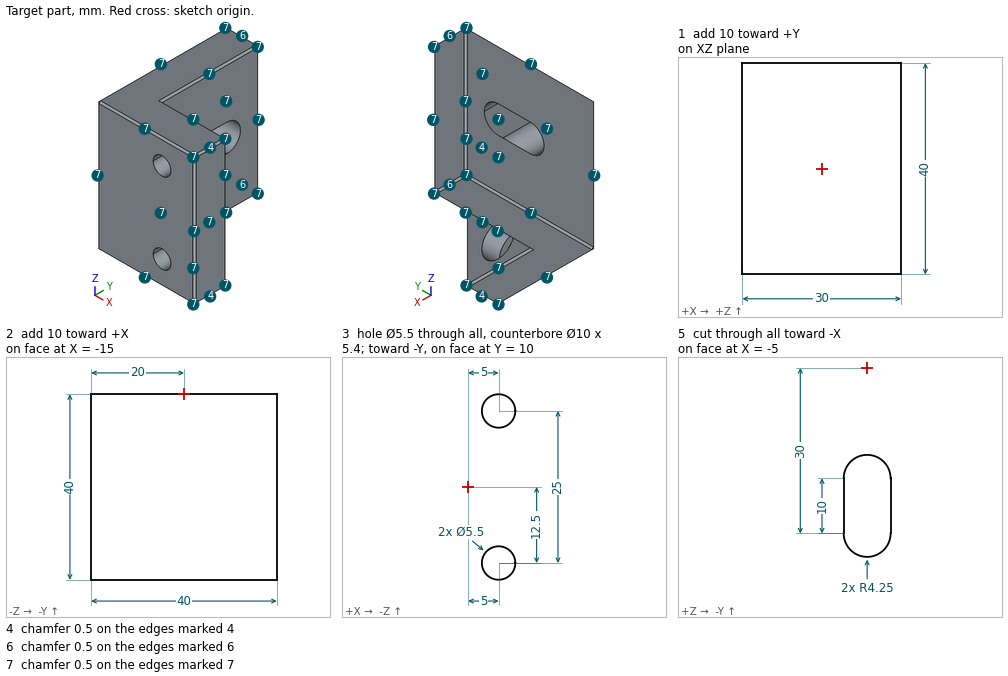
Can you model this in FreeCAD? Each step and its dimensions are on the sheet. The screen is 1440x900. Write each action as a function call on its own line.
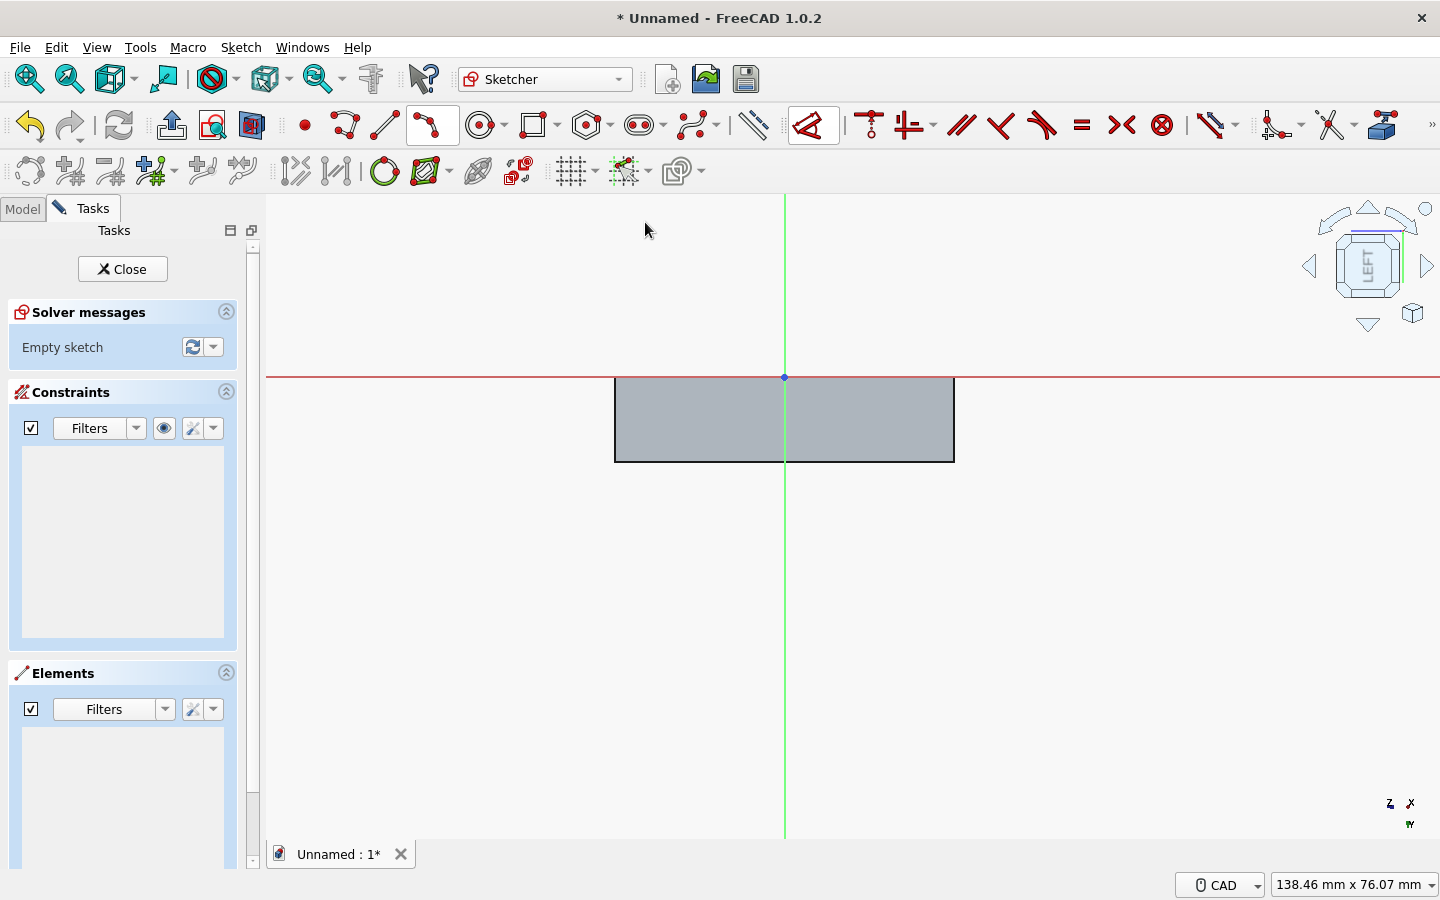
click(534, 126)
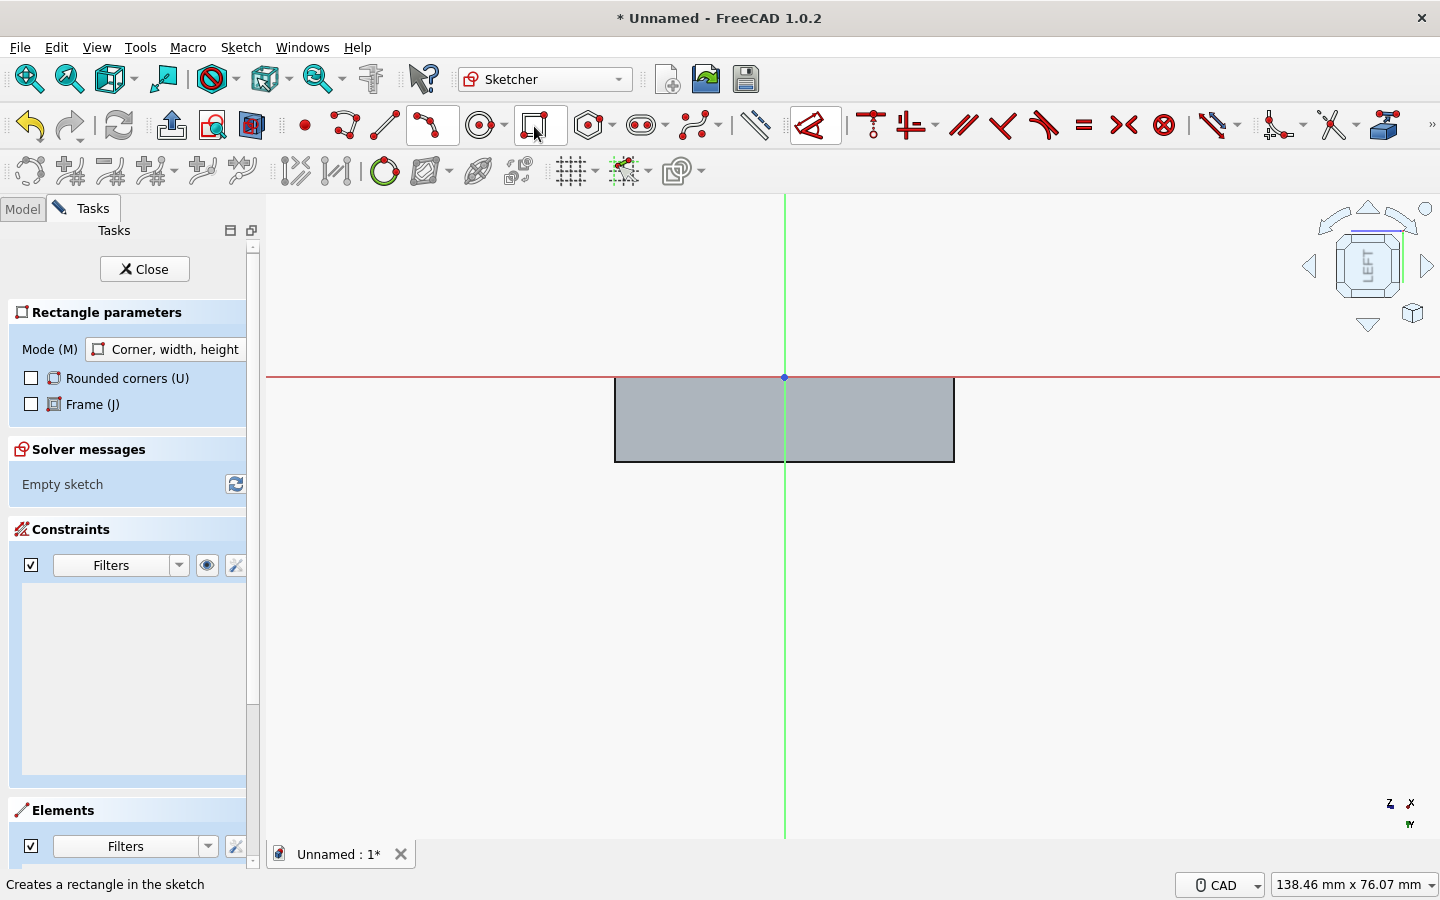
click(615, 377)
click(954, 716)
key(Escape)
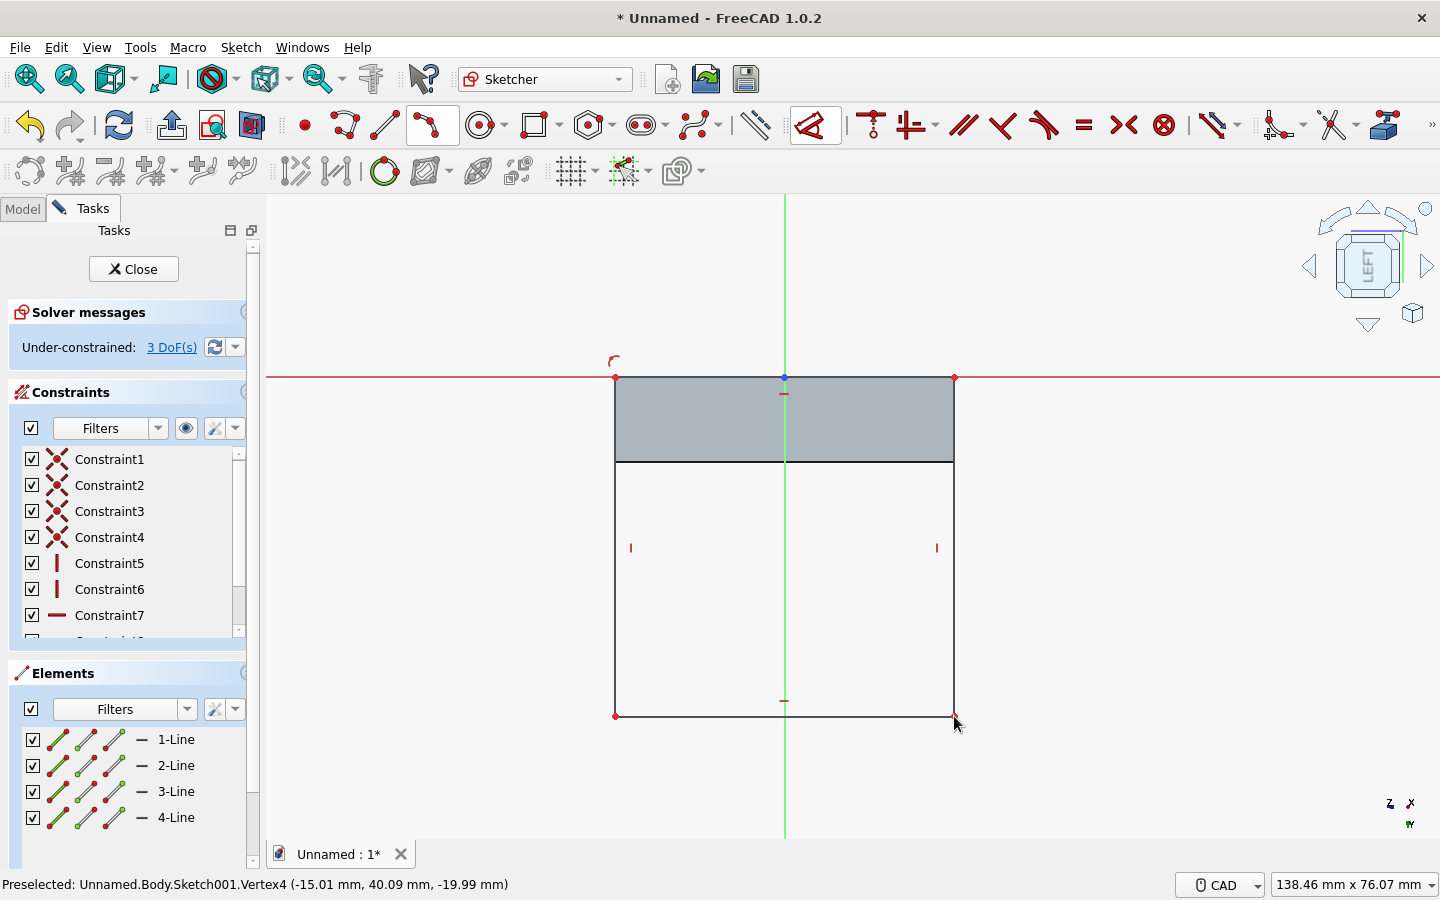
click(615, 479)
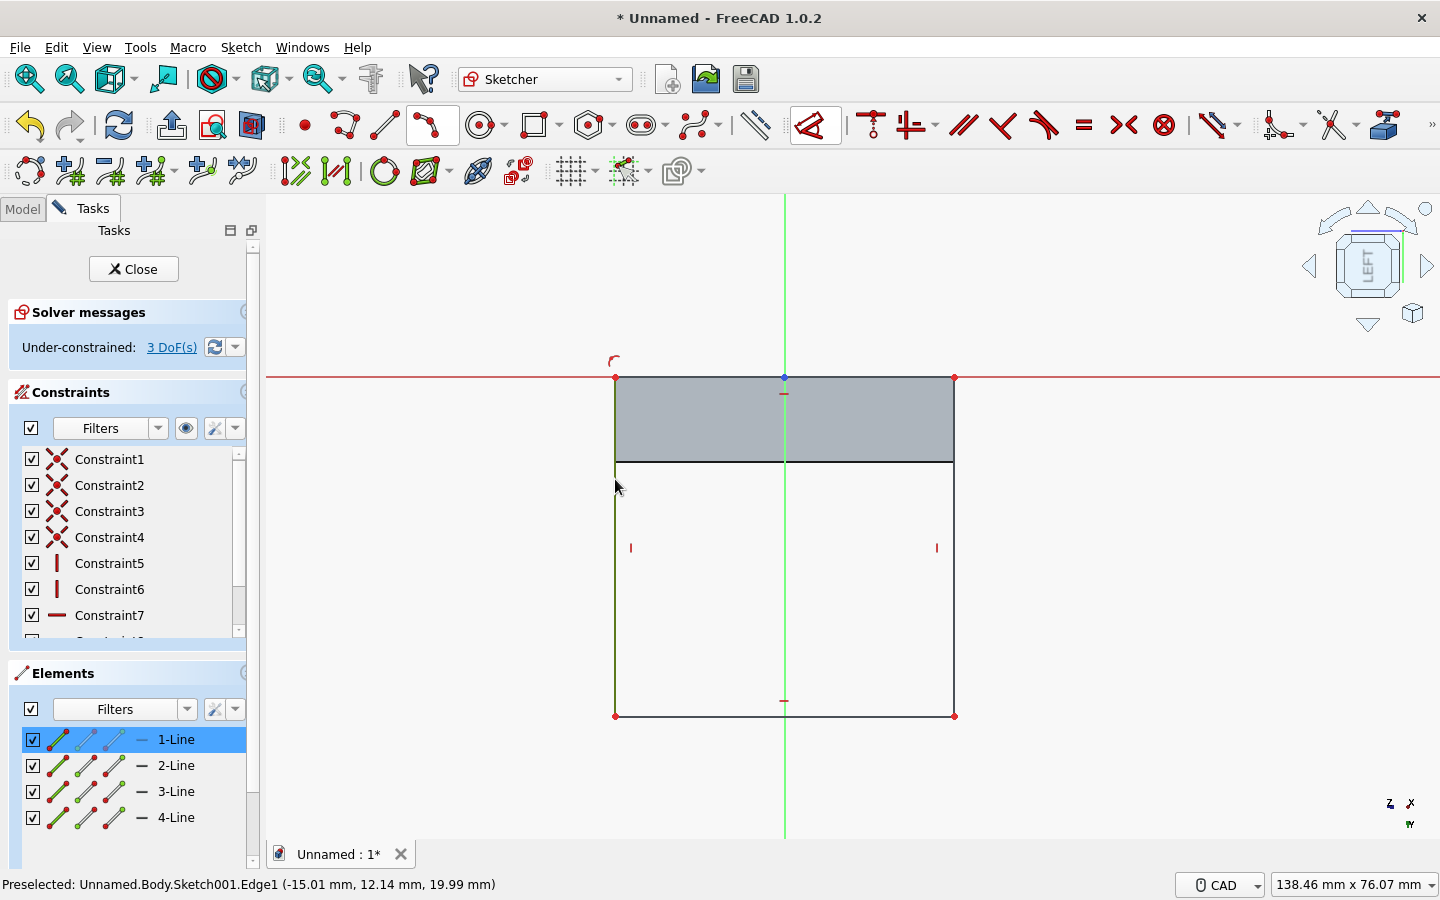
click(836, 126)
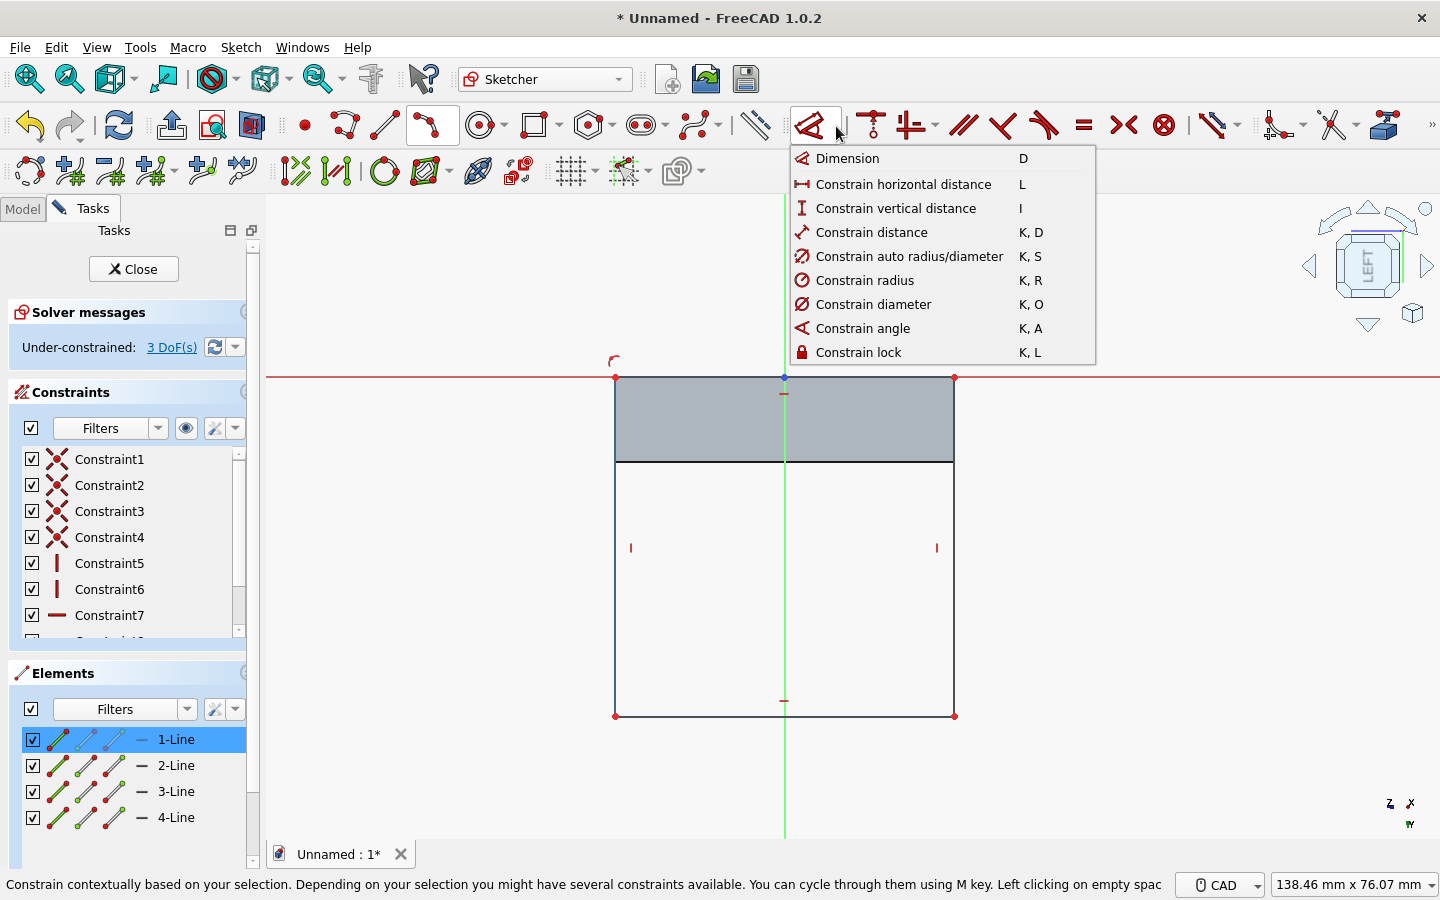
click(943, 208)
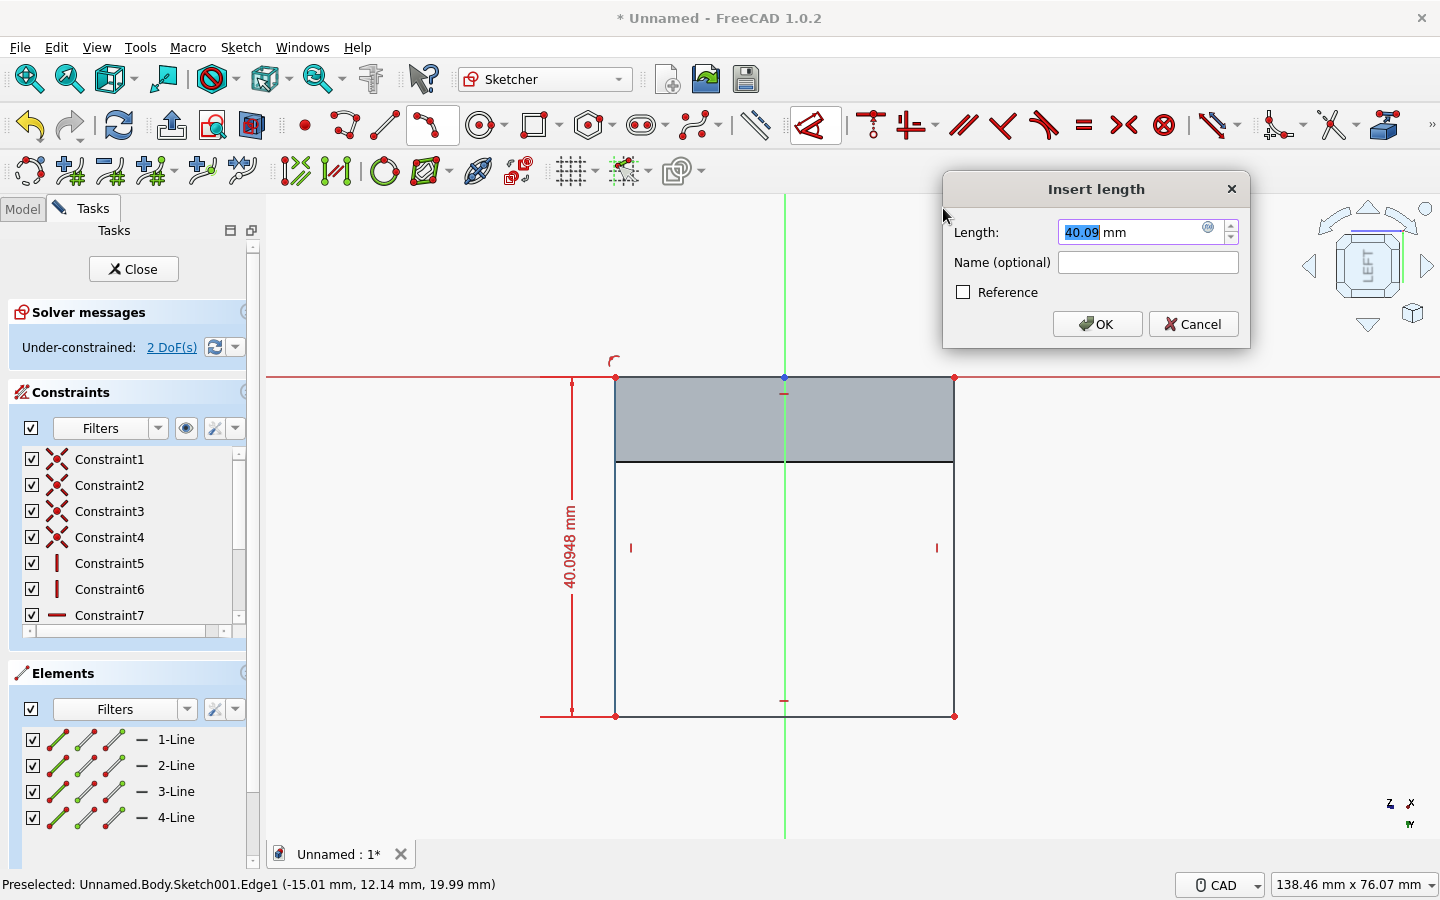
text(40)
key(Return)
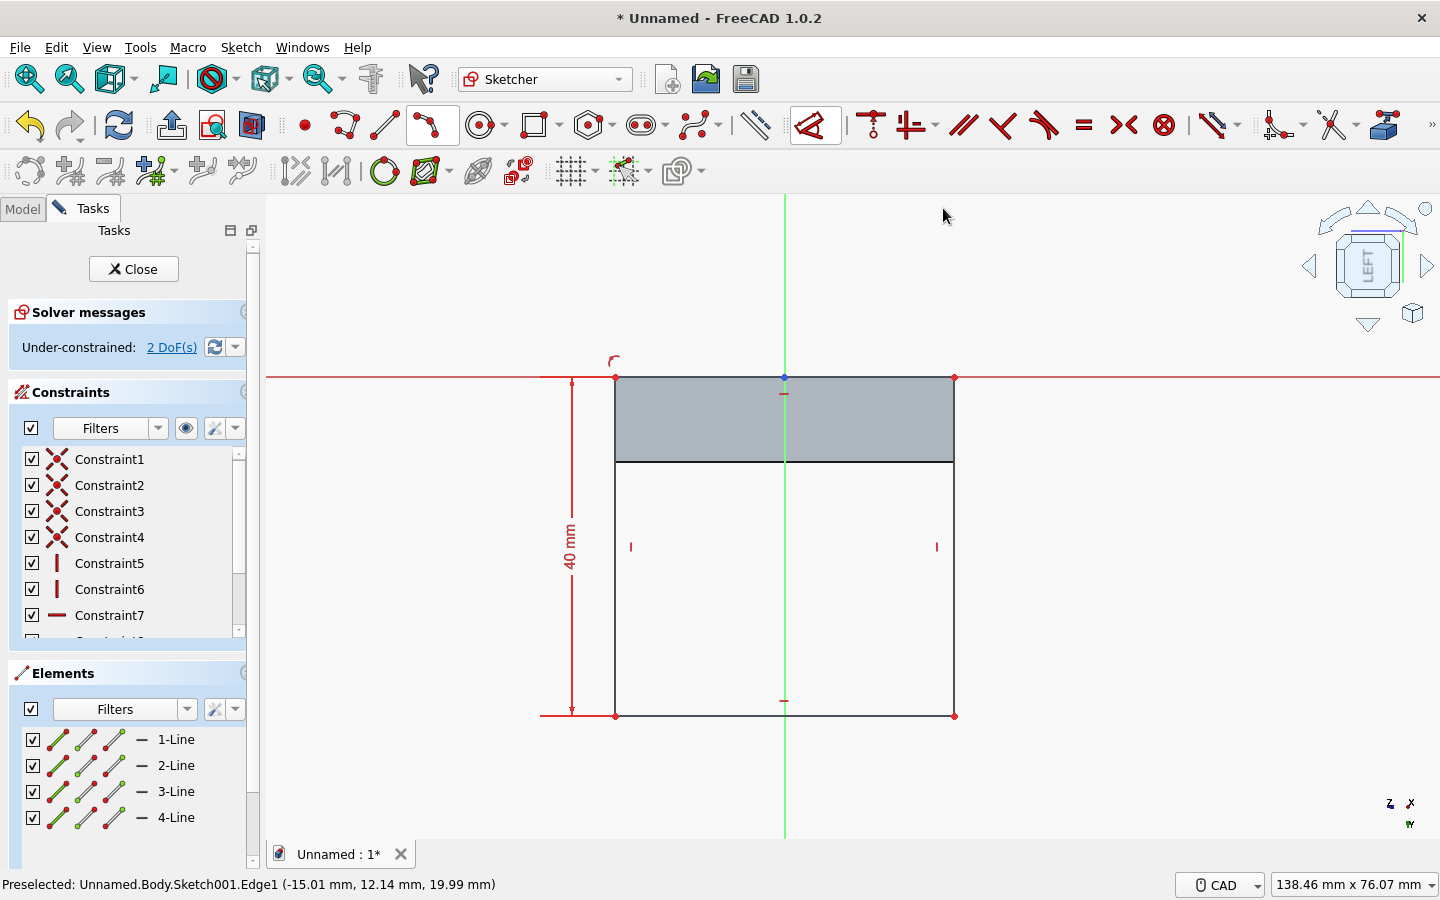
click(717, 716)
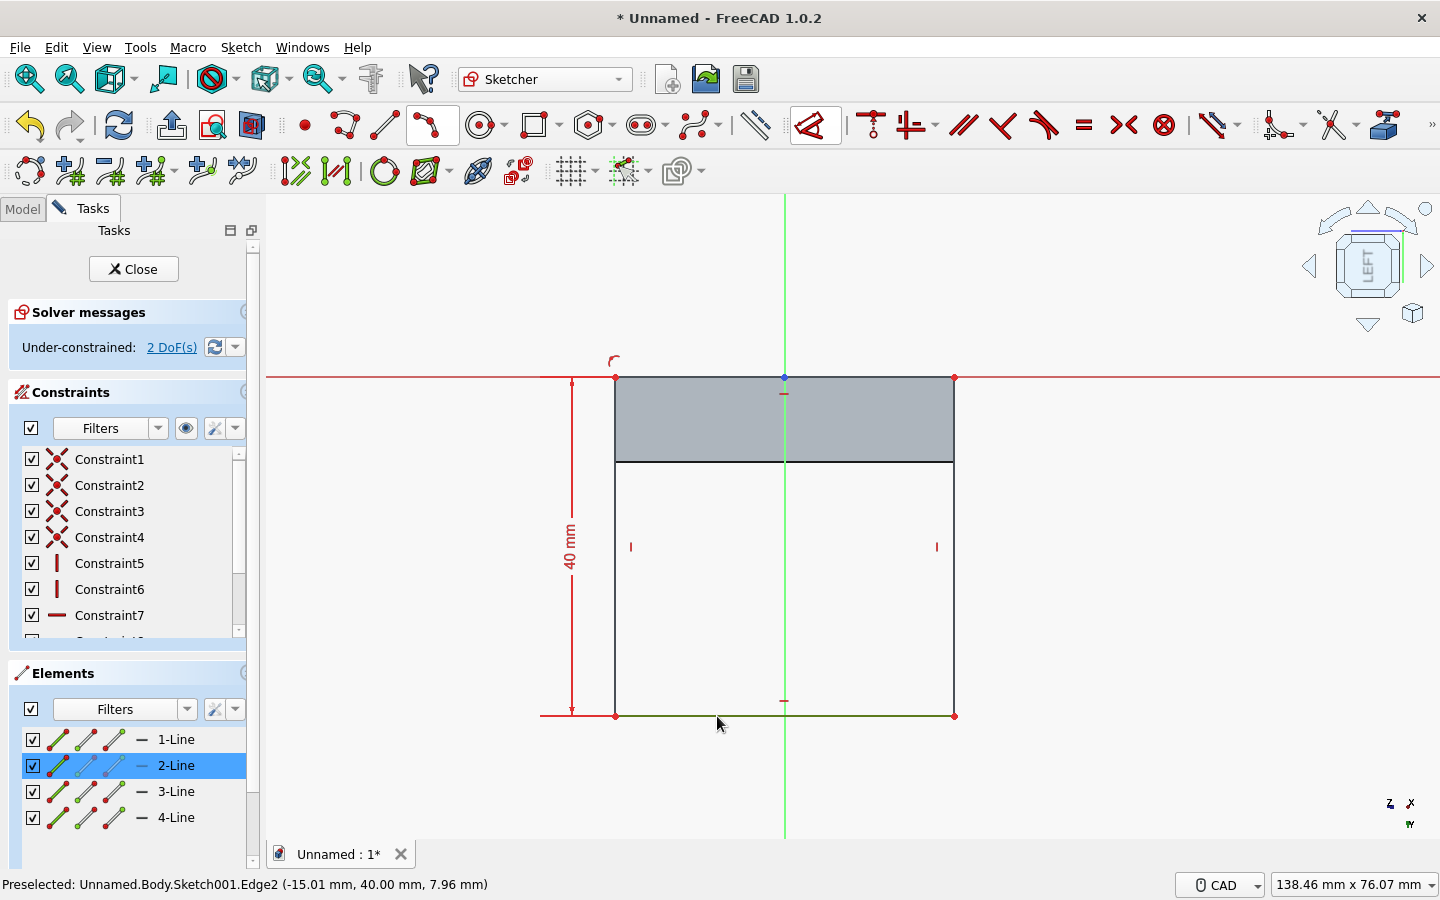
click(836, 126)